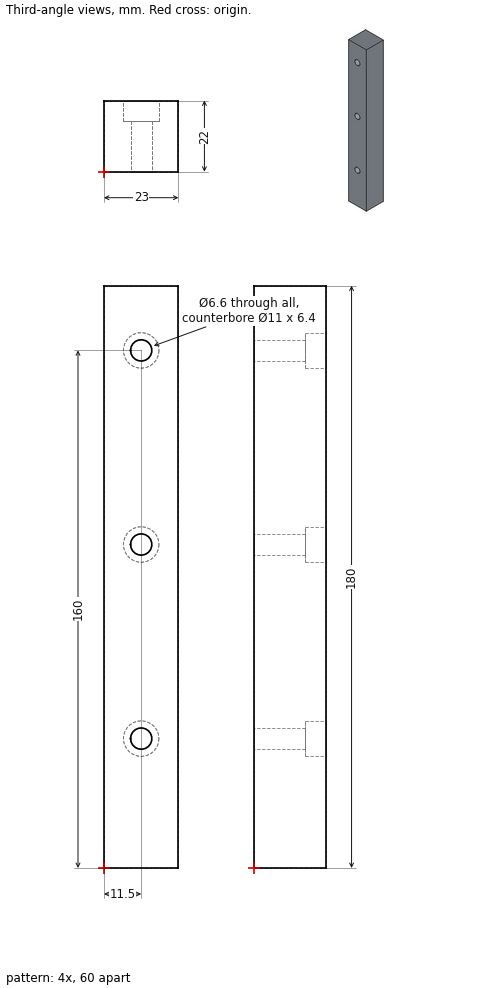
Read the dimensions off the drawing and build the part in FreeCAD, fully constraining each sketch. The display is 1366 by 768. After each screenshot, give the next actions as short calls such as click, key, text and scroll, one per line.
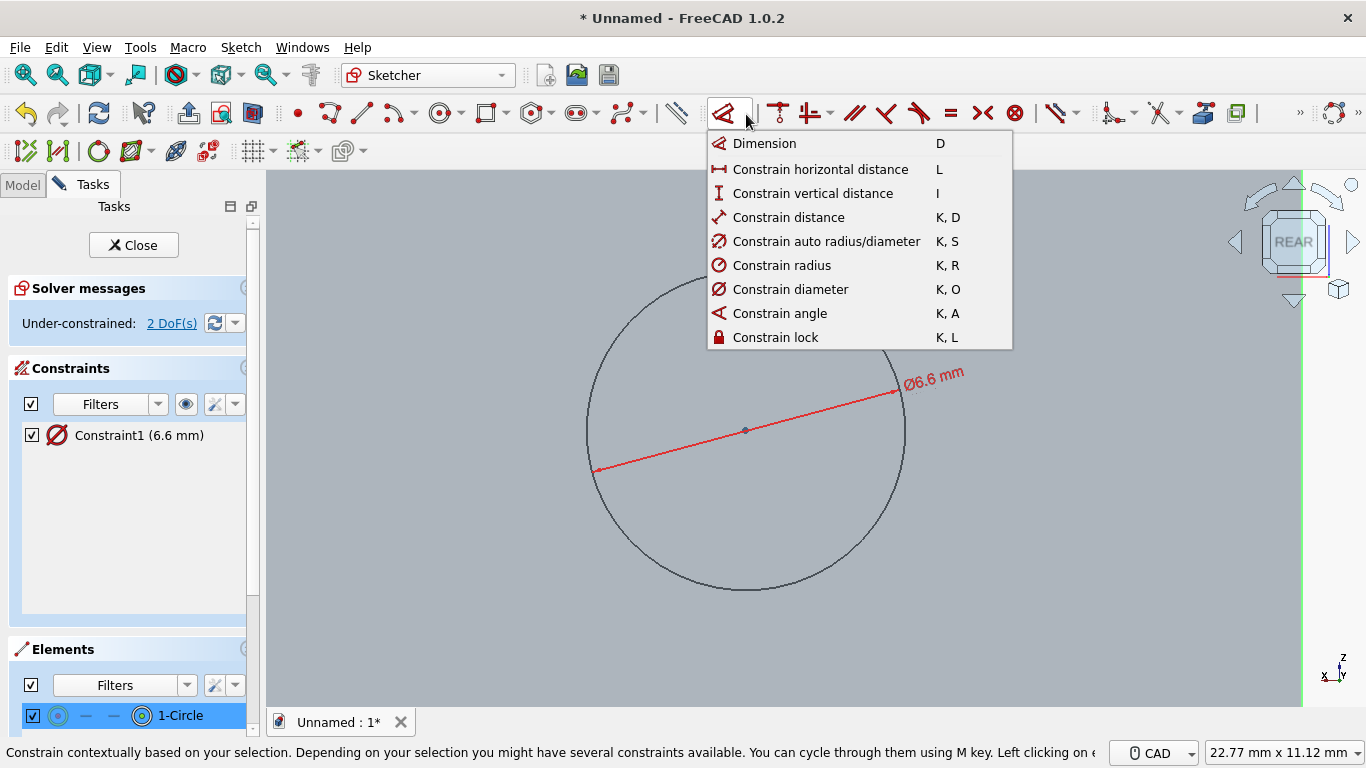
click(860, 193)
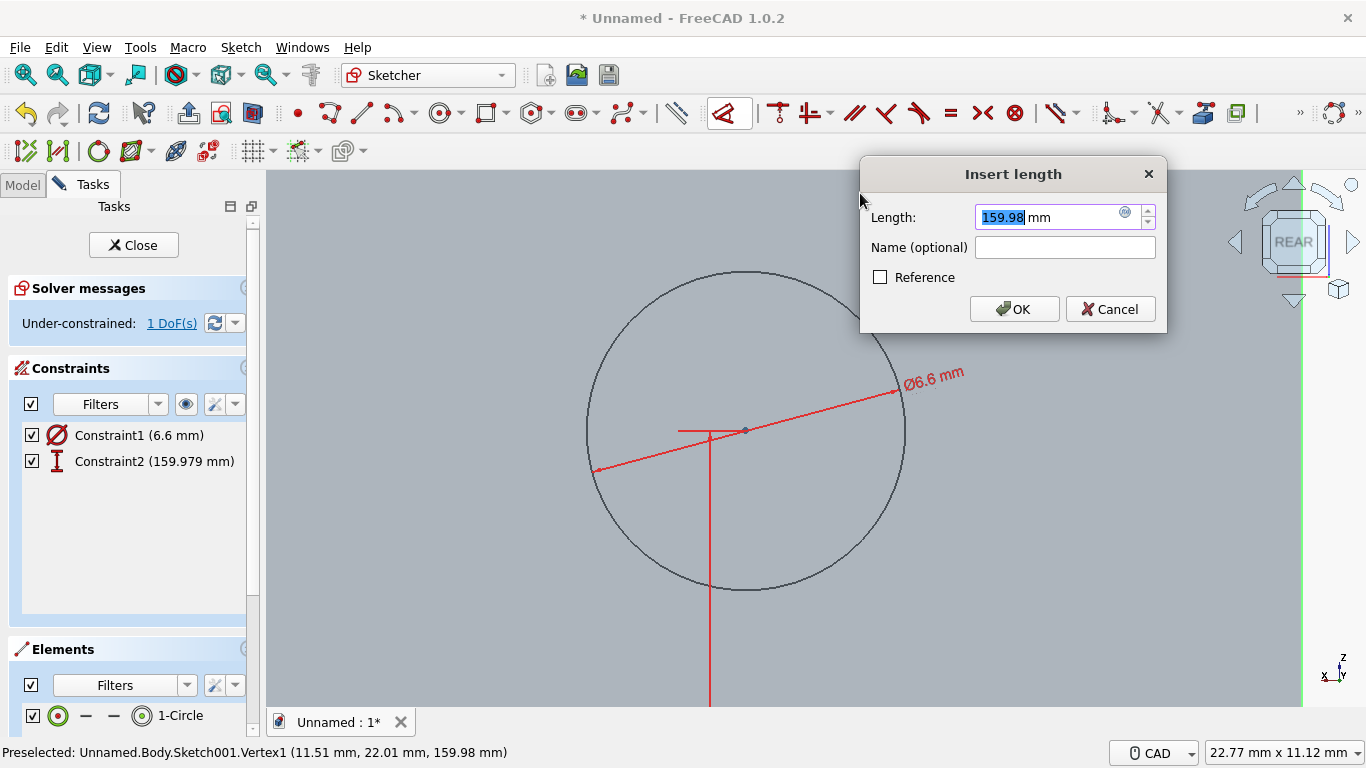
text(160)
key(Return)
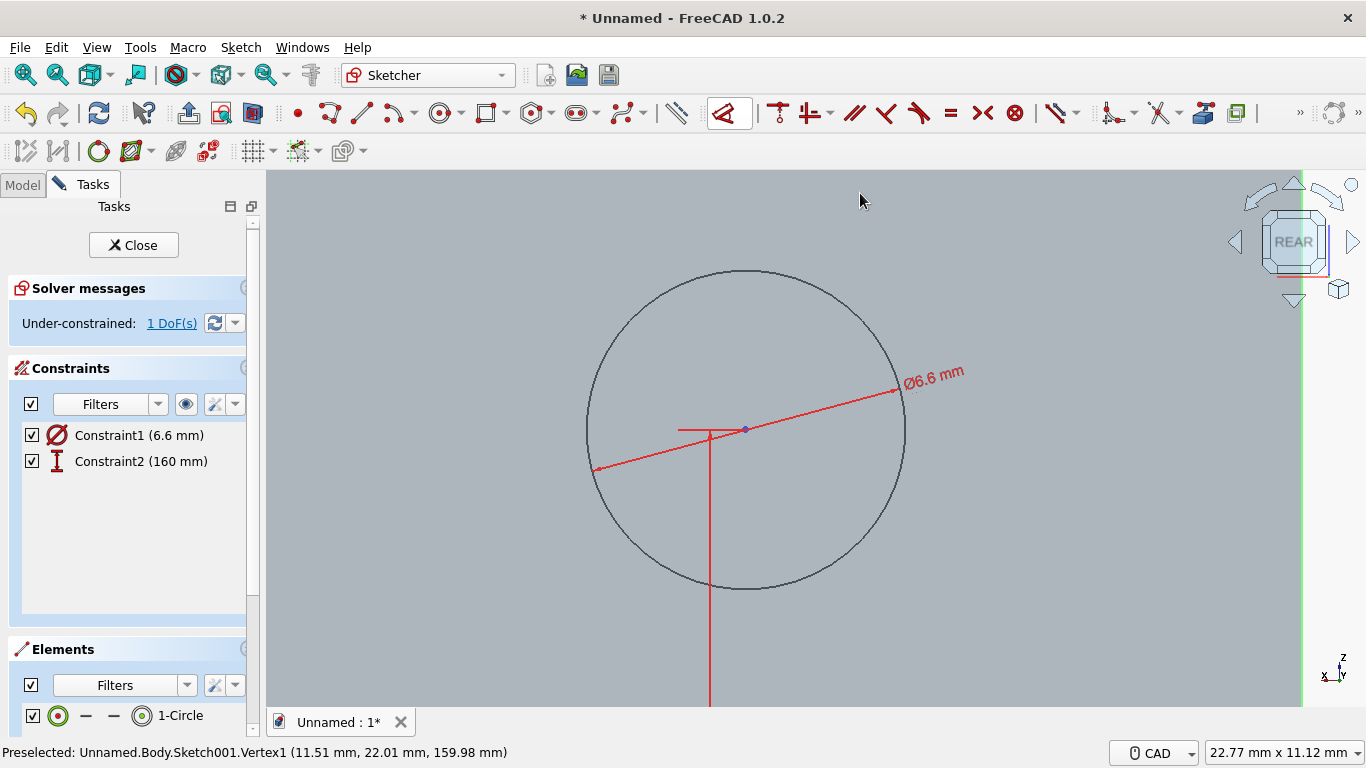
click(746, 430)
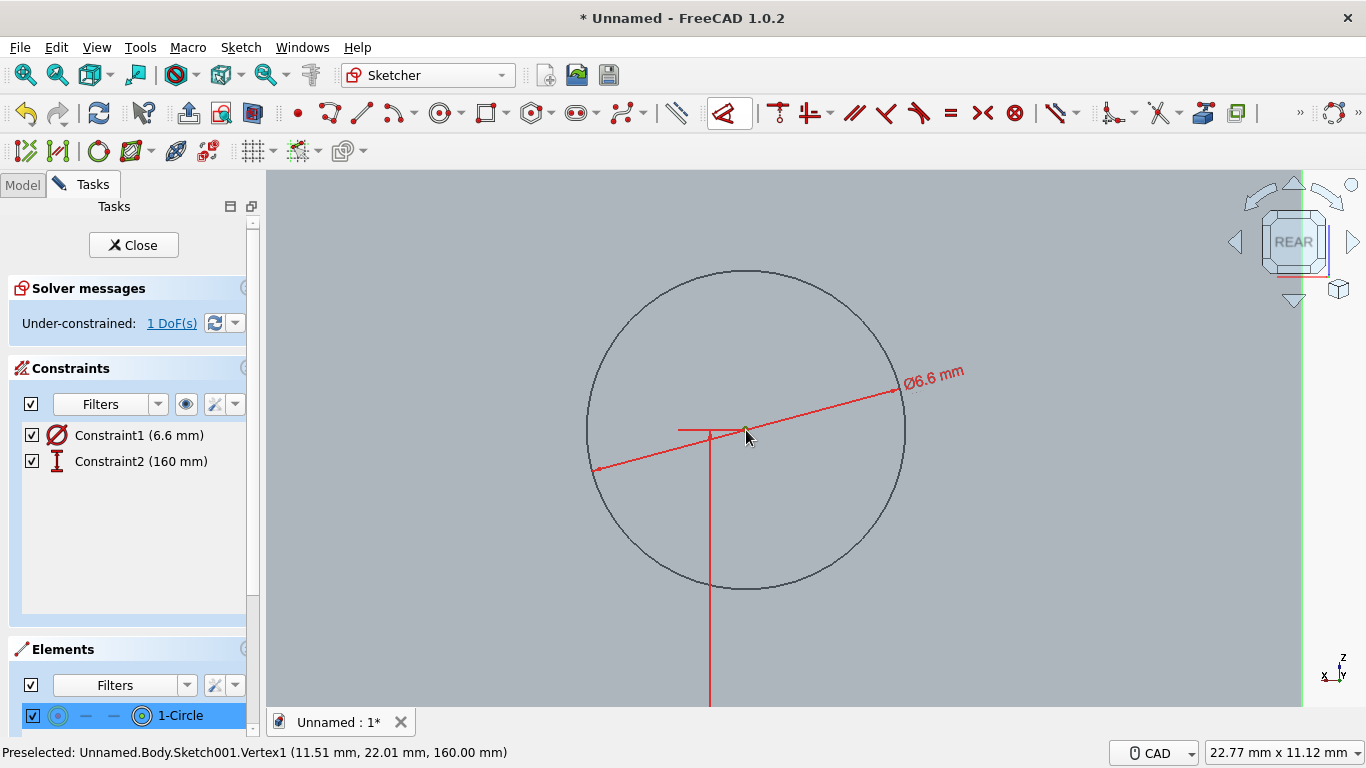
key(l)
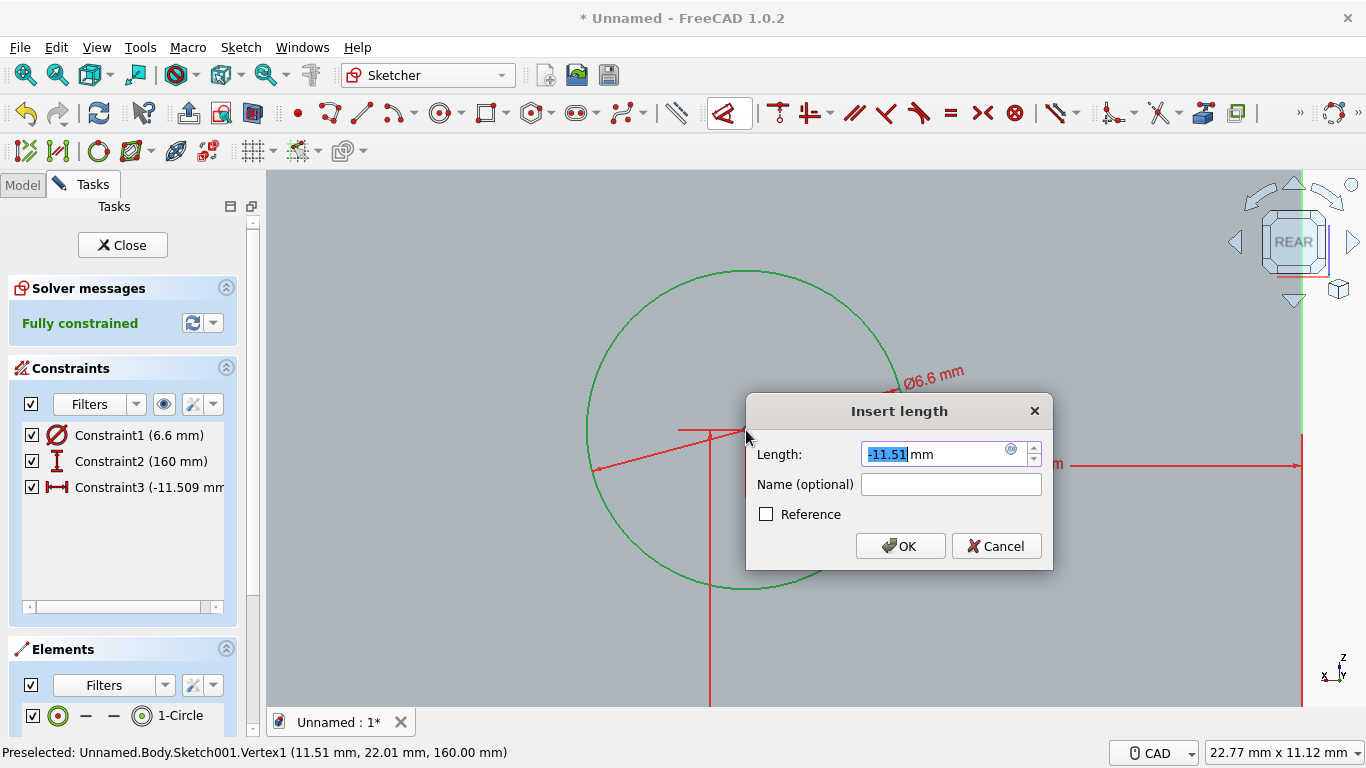
text(-11.5)
key(Return)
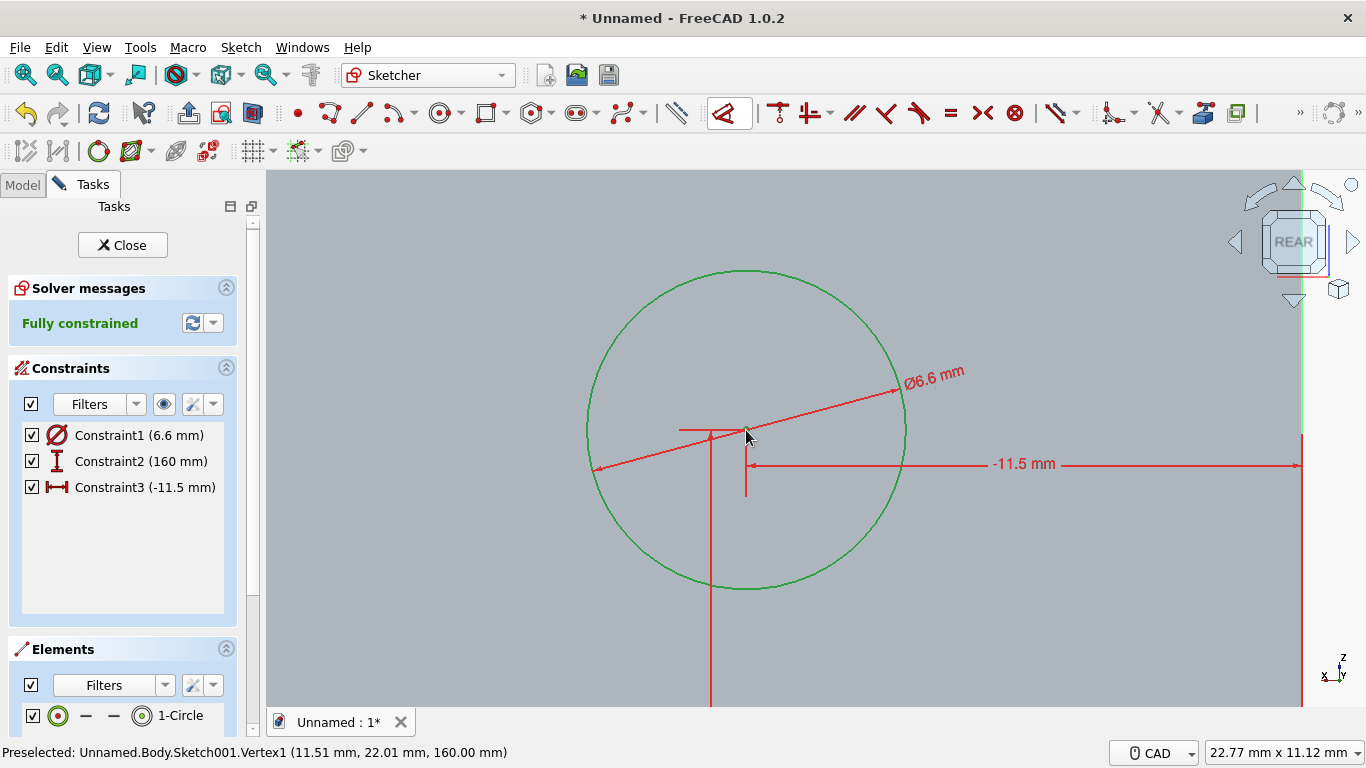
click(123, 245)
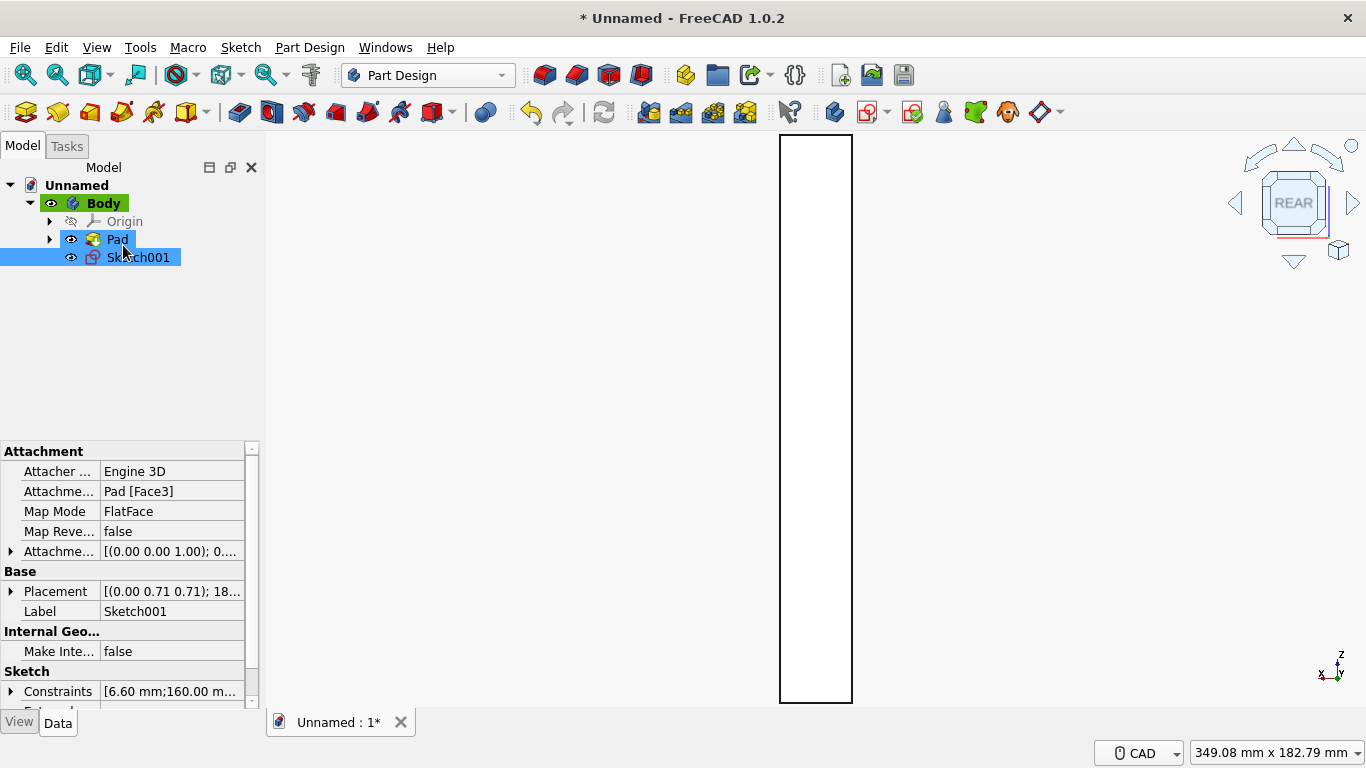
click(272, 112)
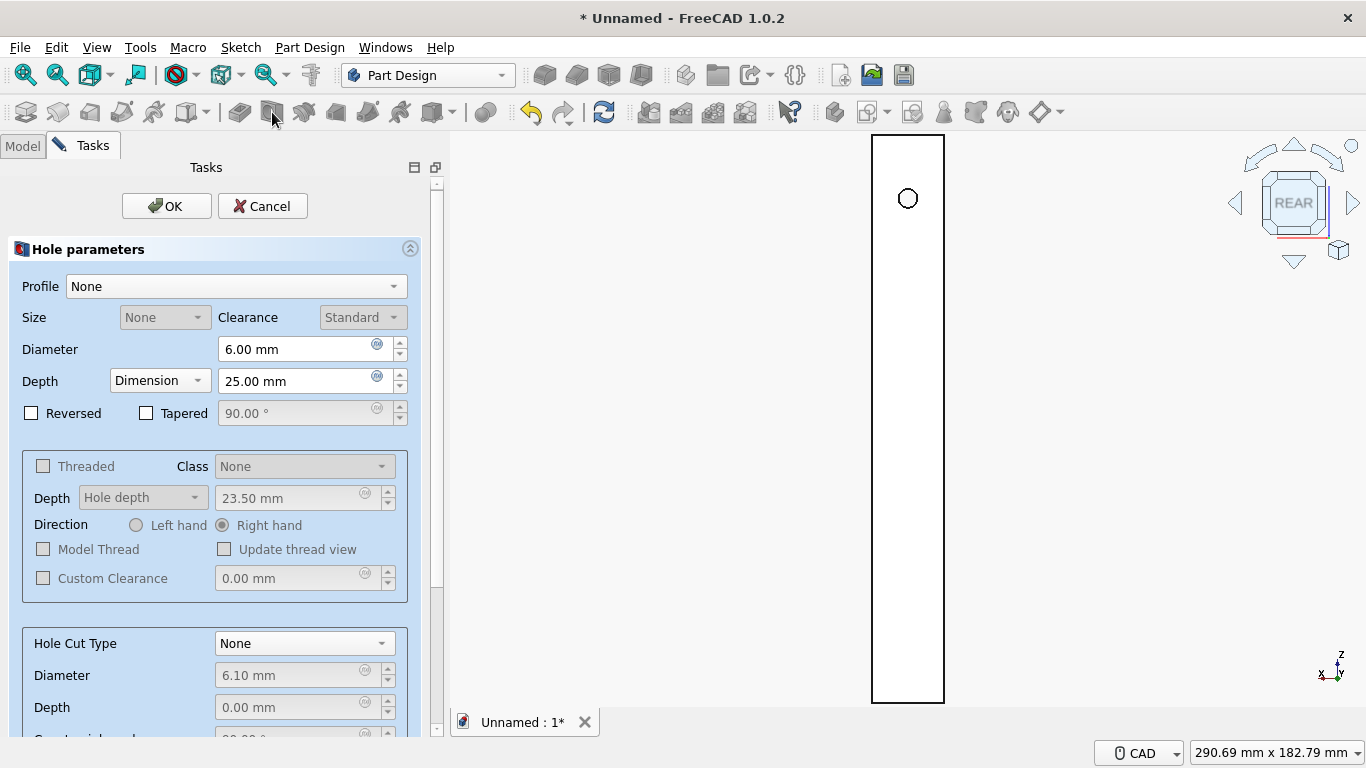
triple_click(305, 349)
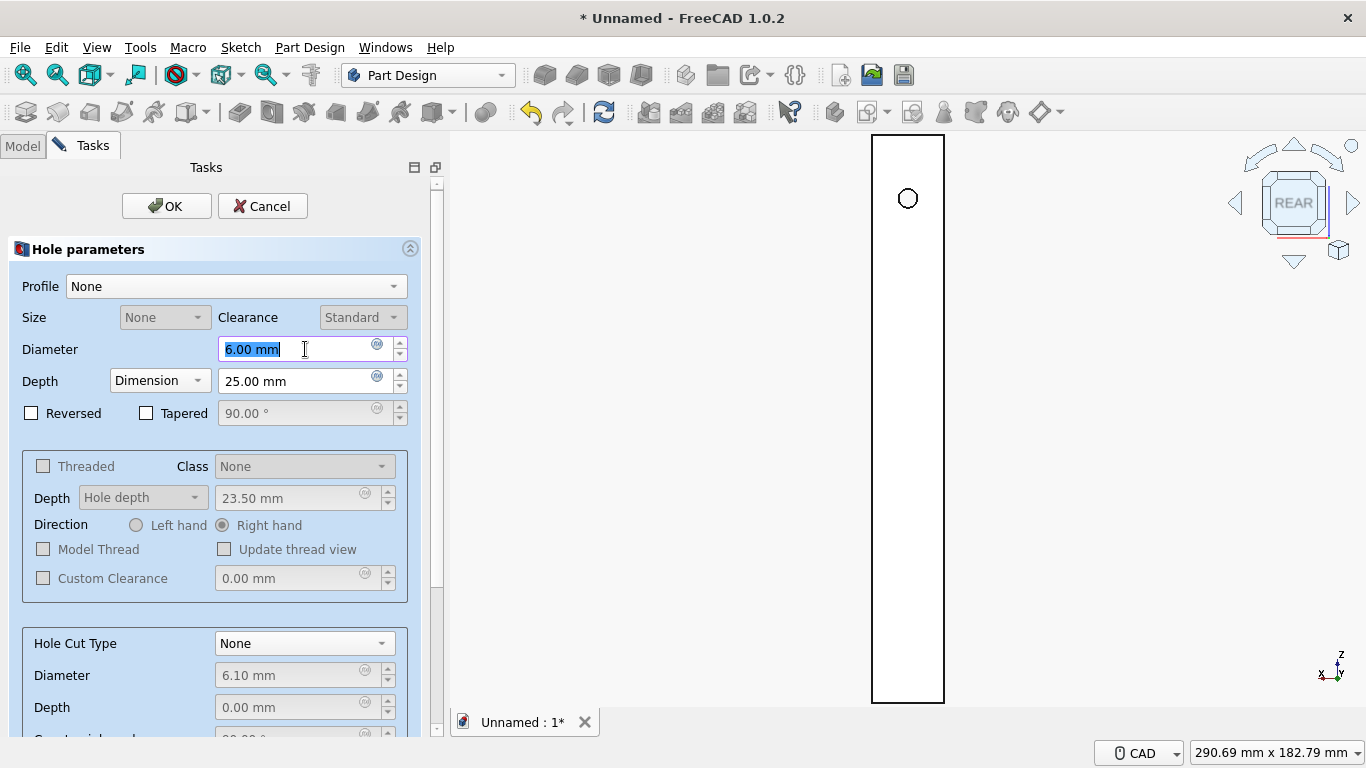
text(6.6)
key(Tab)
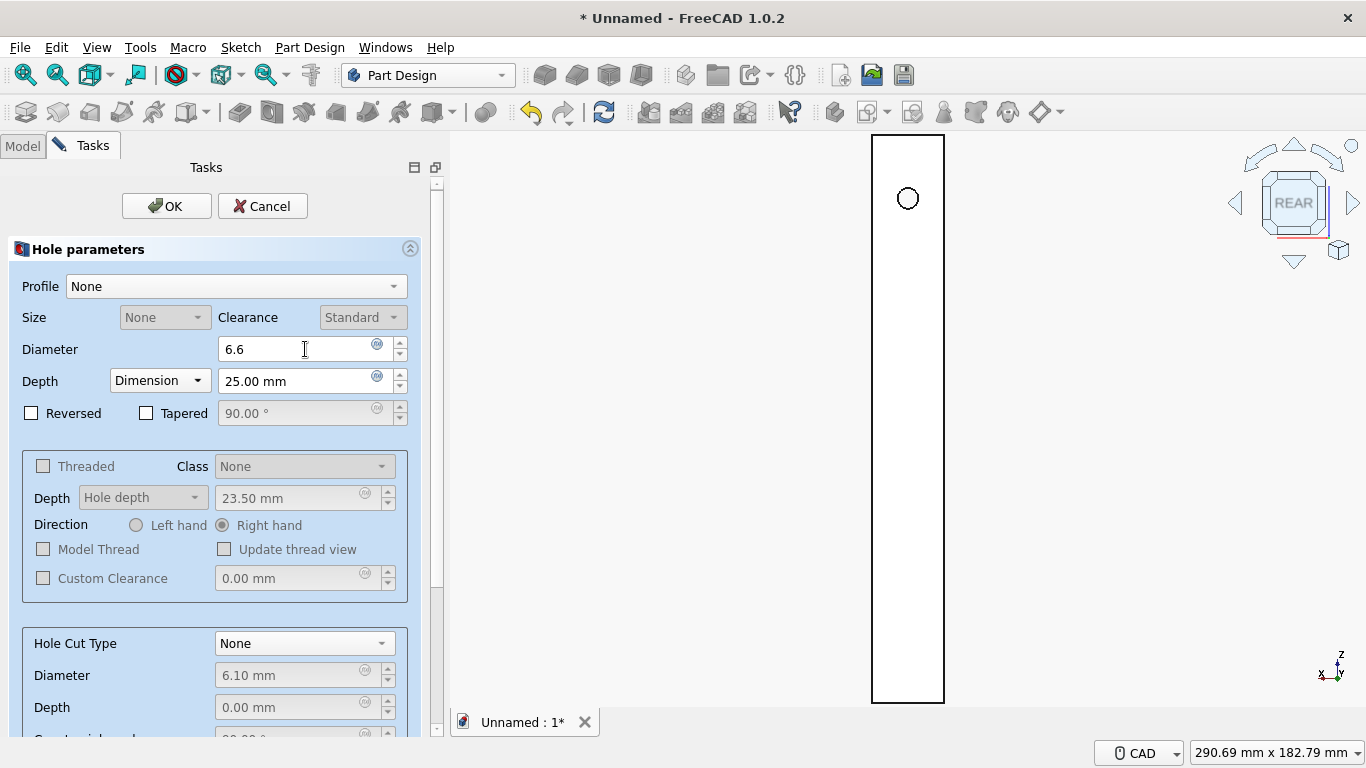
click(161, 380)